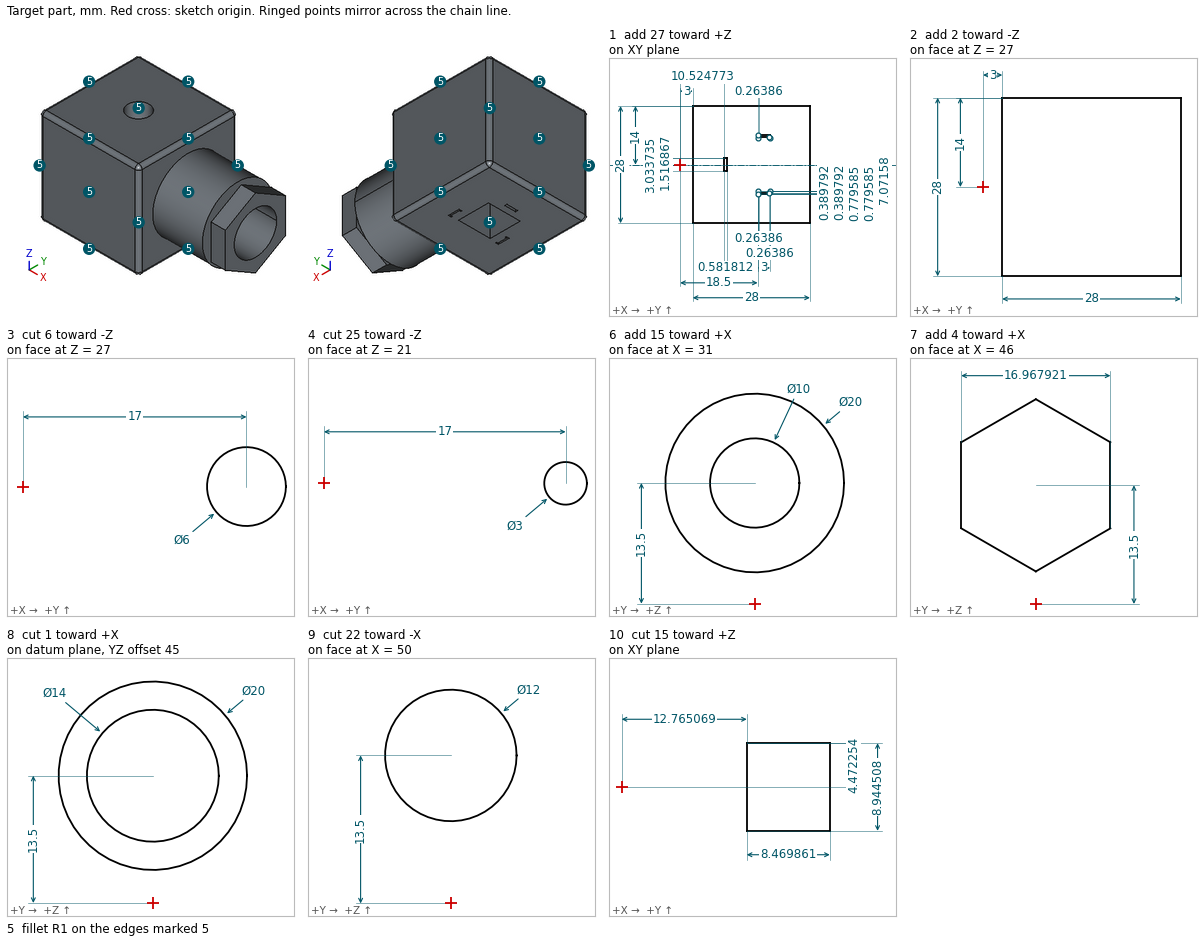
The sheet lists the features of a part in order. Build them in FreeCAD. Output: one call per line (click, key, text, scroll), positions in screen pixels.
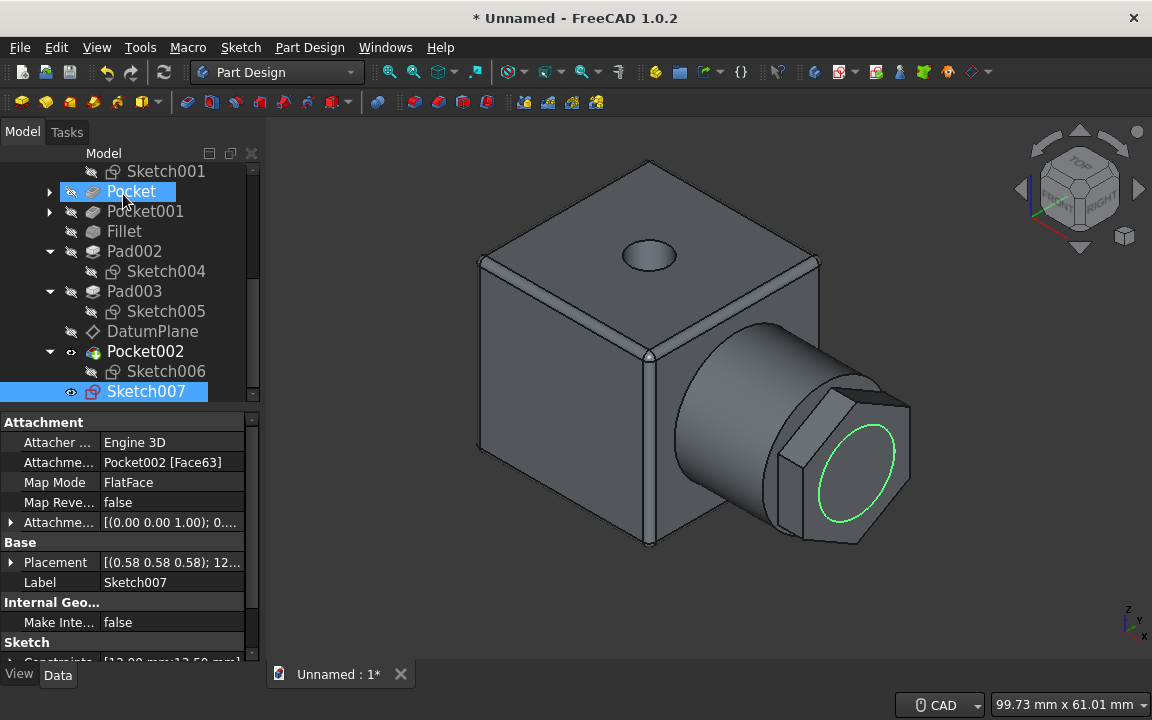
click(188, 102)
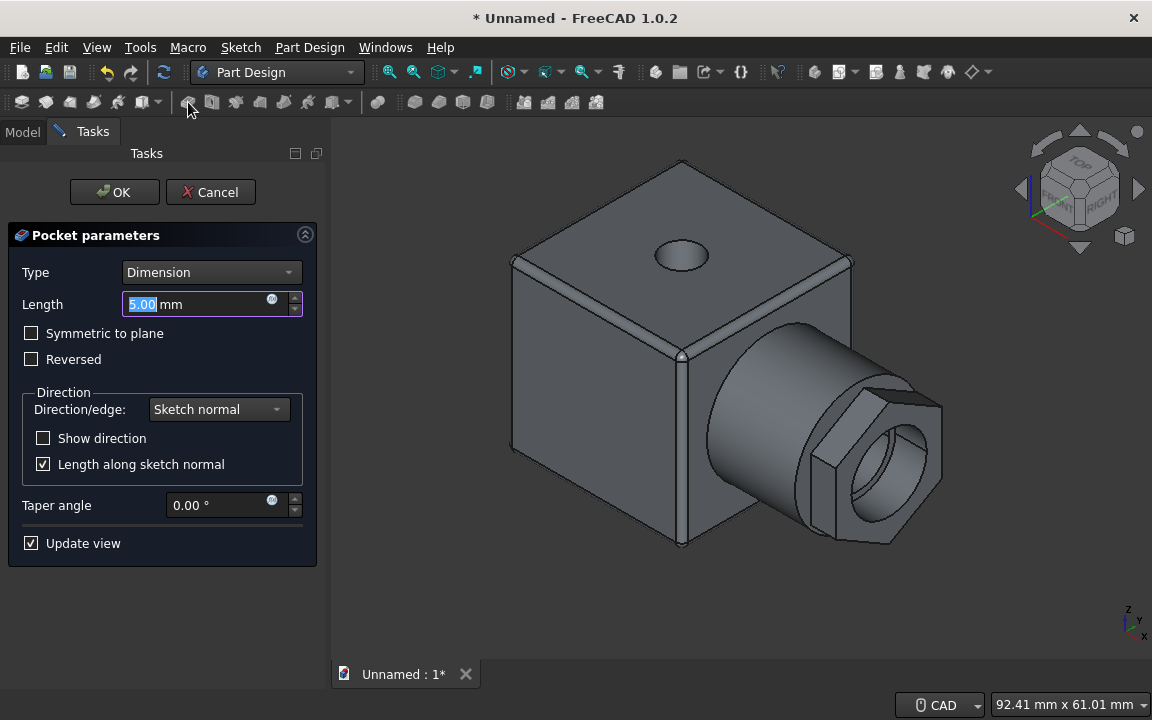
text(22)
key(Tab)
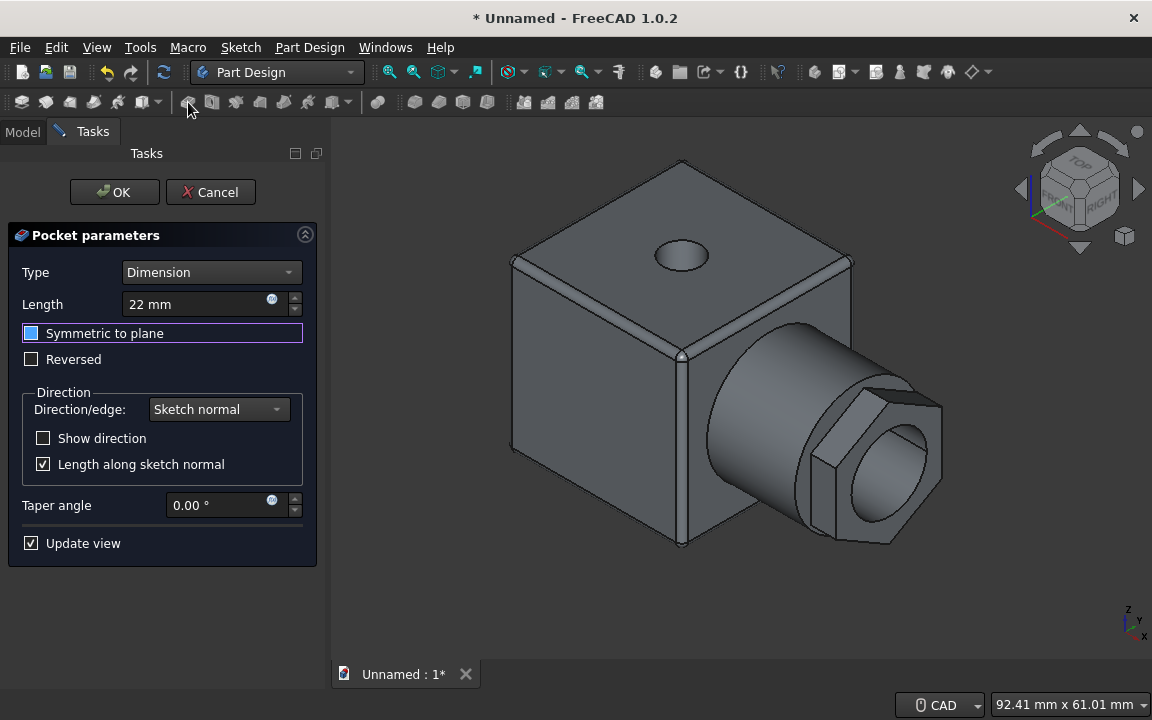
click(115, 192)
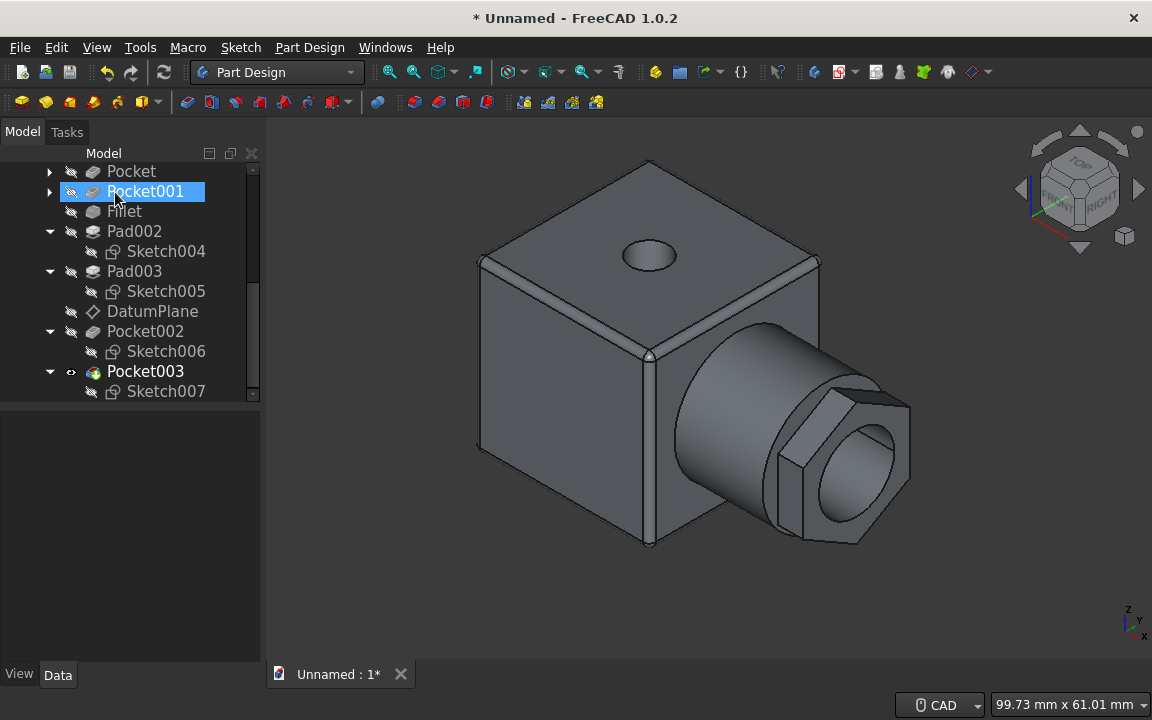
click(840, 72)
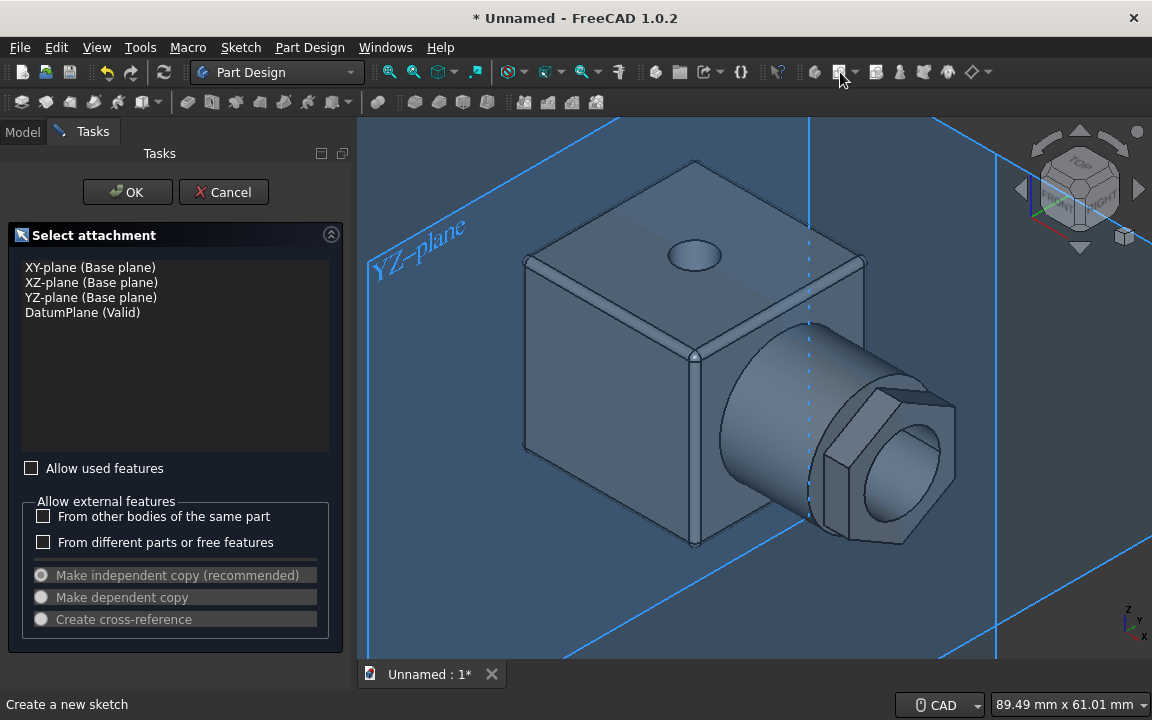
click(82, 268)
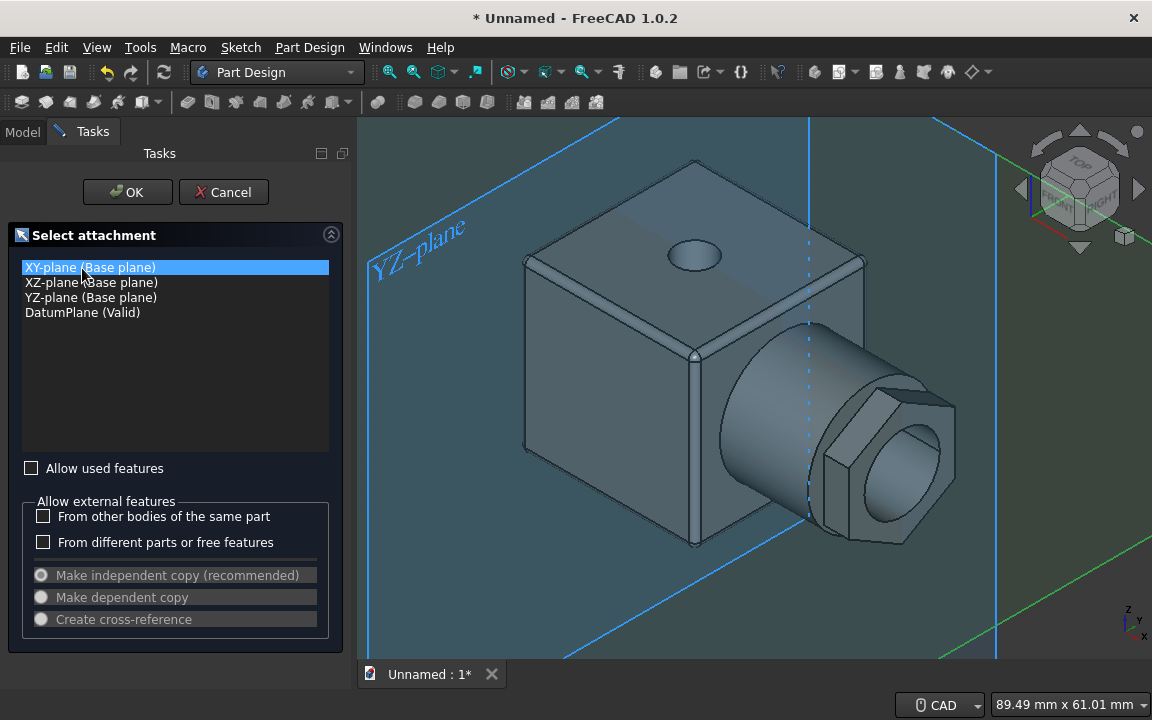
click(128, 192)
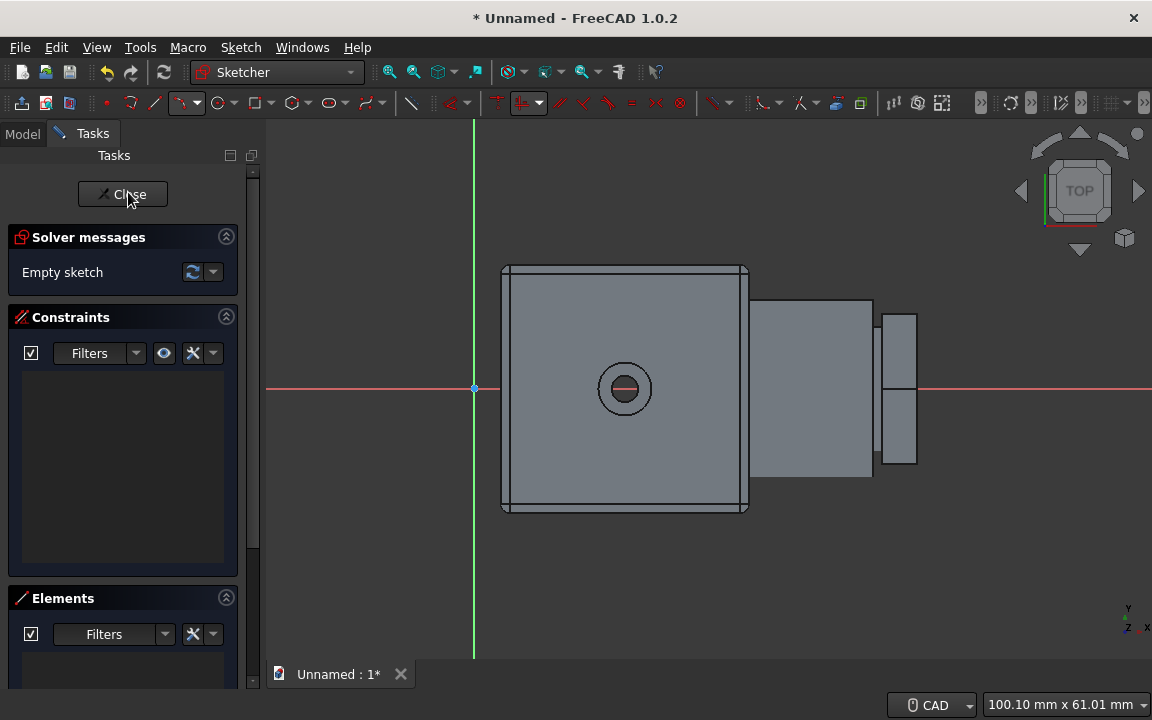
click(70, 104)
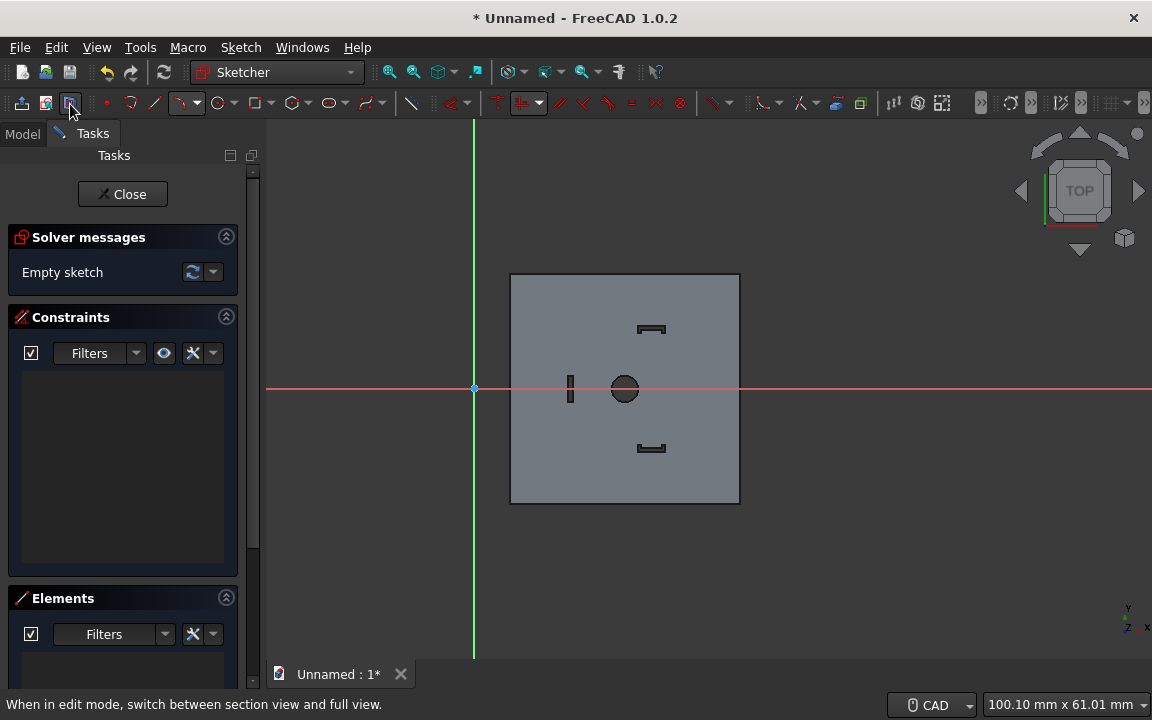
scroll(526, 389, up, 5)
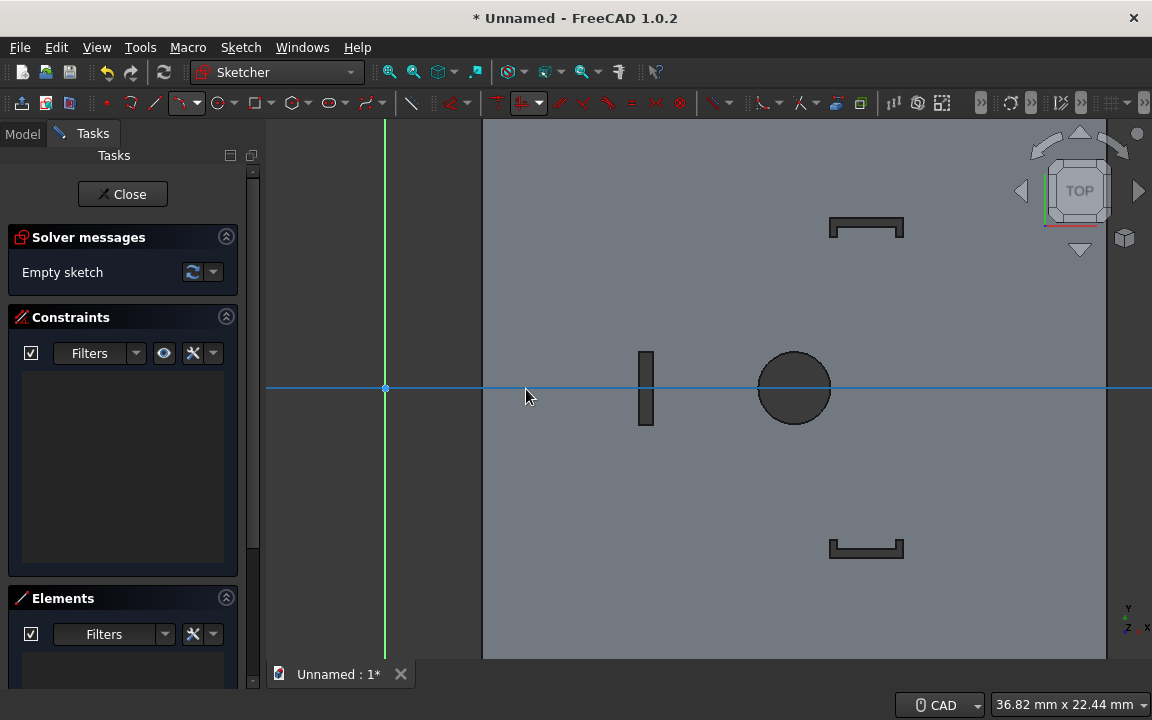
click(256, 104)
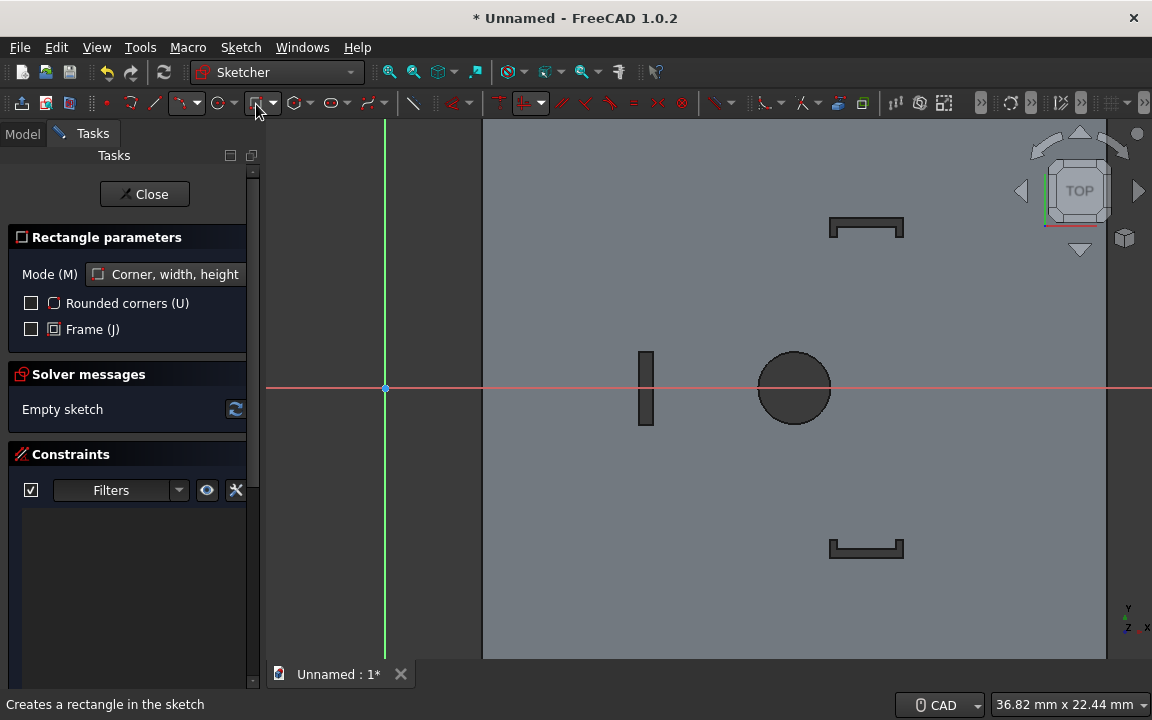
click(692, 281)
click(896, 496)
key(Escape)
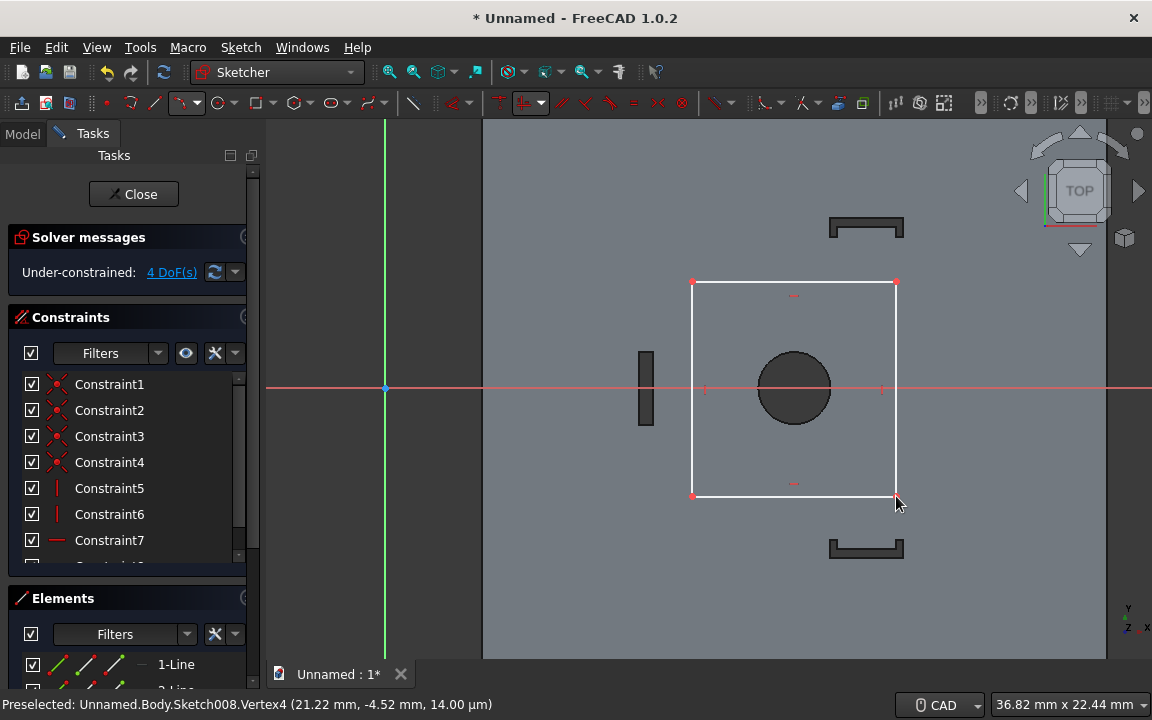
click(452, 104)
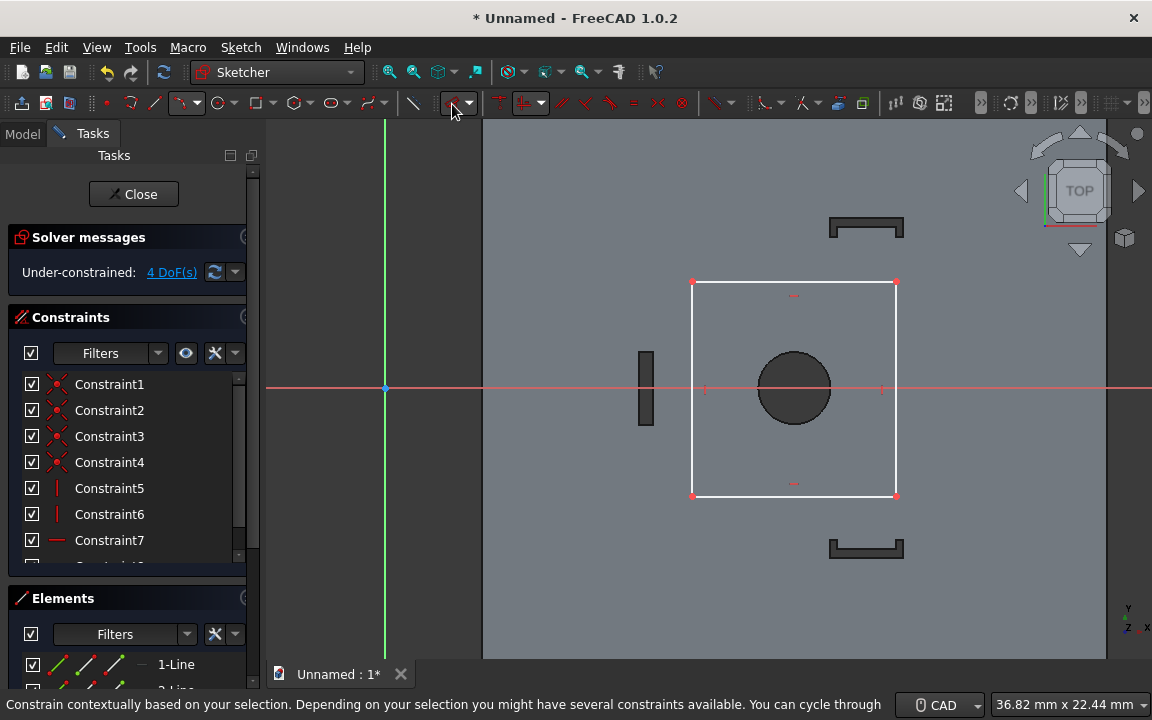
click(692, 347)
click(726, 340)